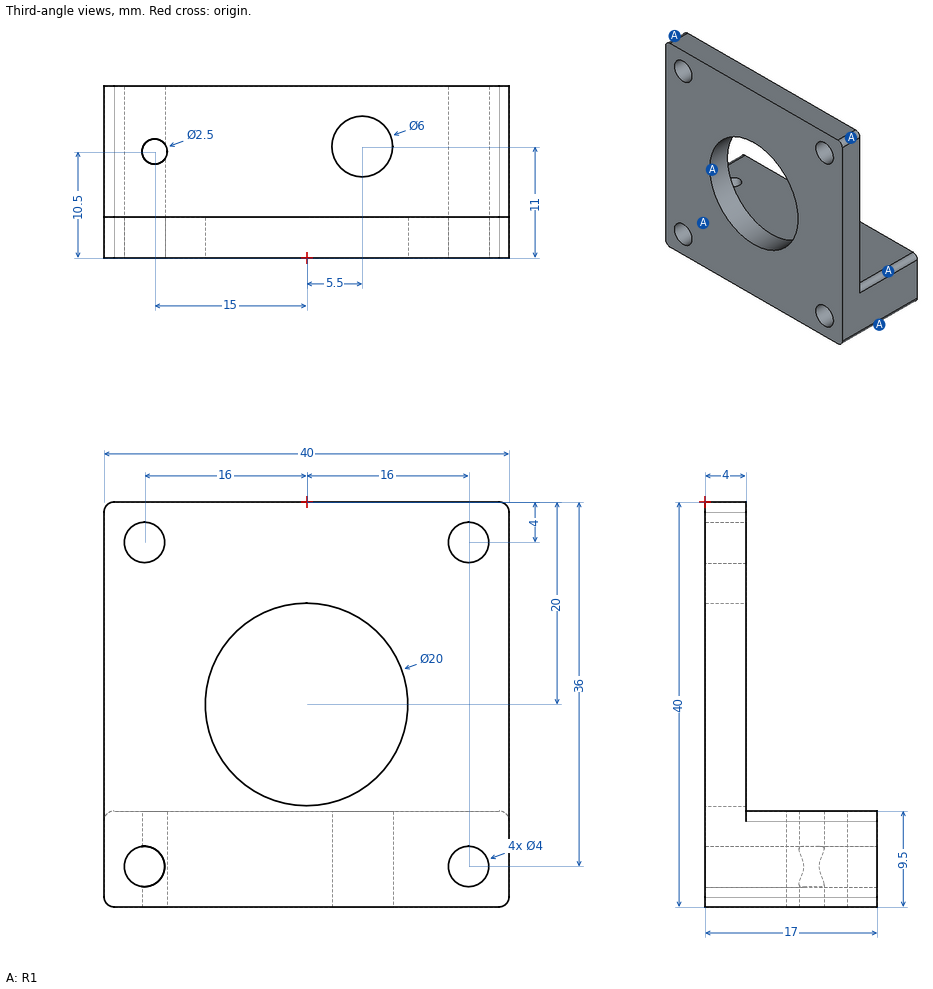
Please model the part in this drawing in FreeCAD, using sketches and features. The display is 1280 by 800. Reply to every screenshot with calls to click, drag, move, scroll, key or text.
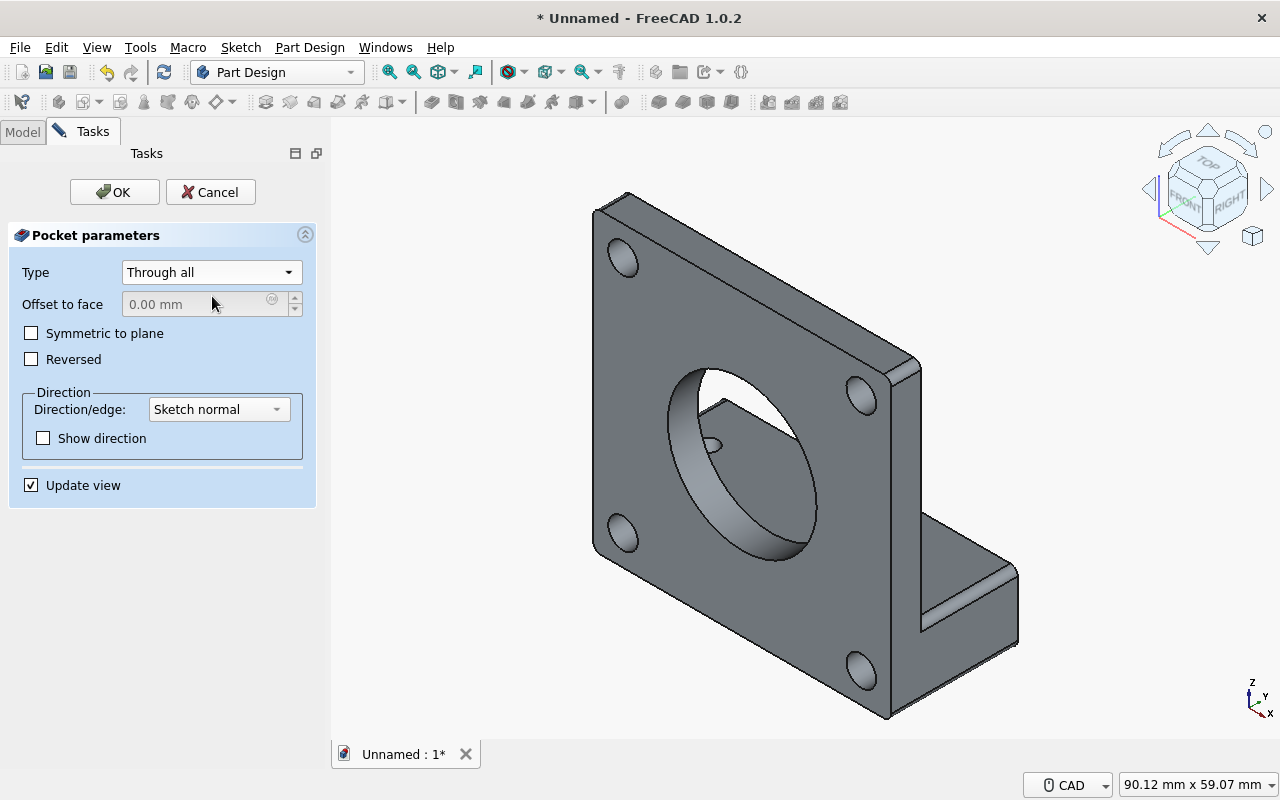
click(115, 192)